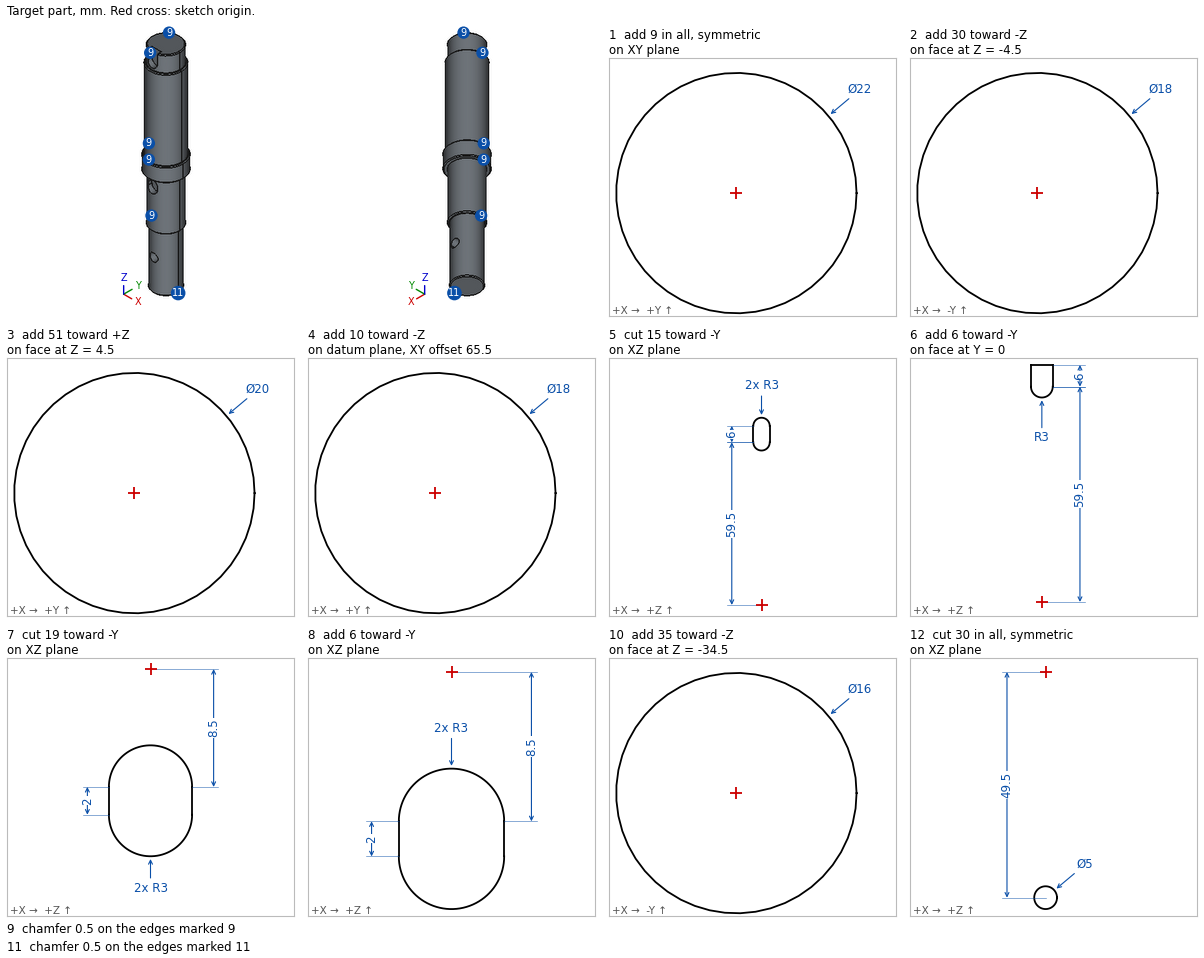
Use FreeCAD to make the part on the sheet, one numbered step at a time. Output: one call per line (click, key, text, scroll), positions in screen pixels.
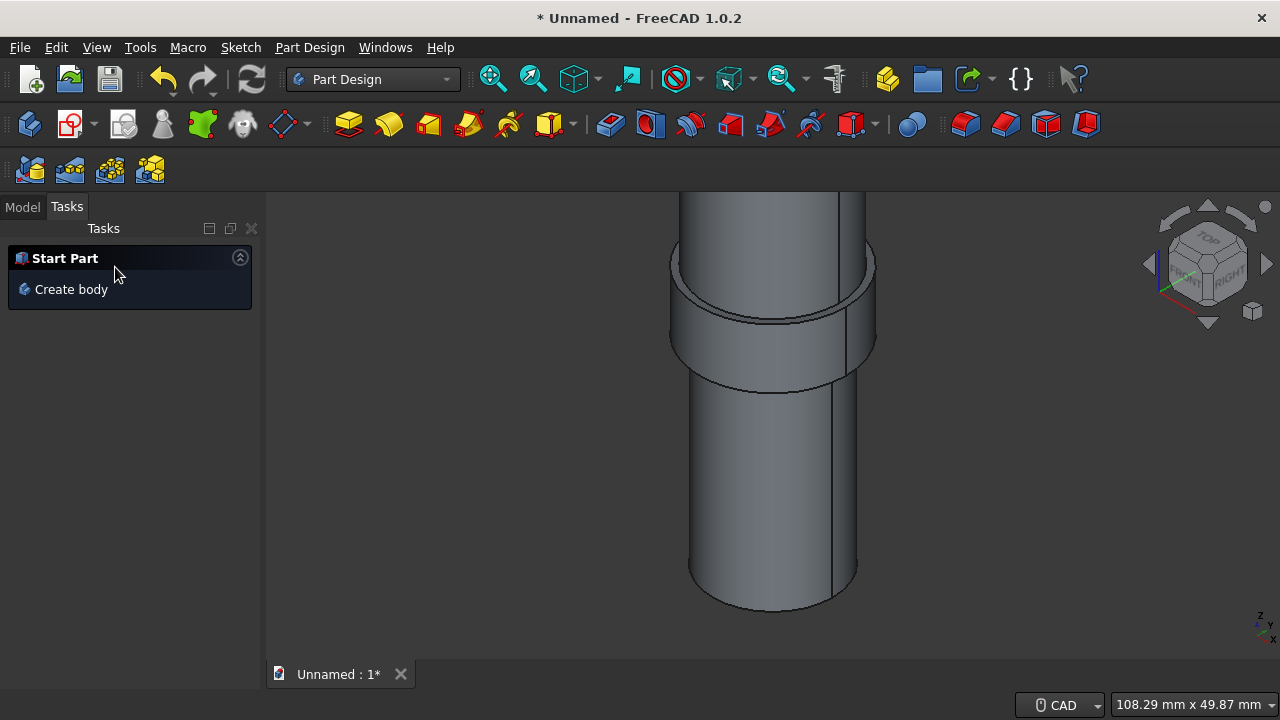
click(494, 80)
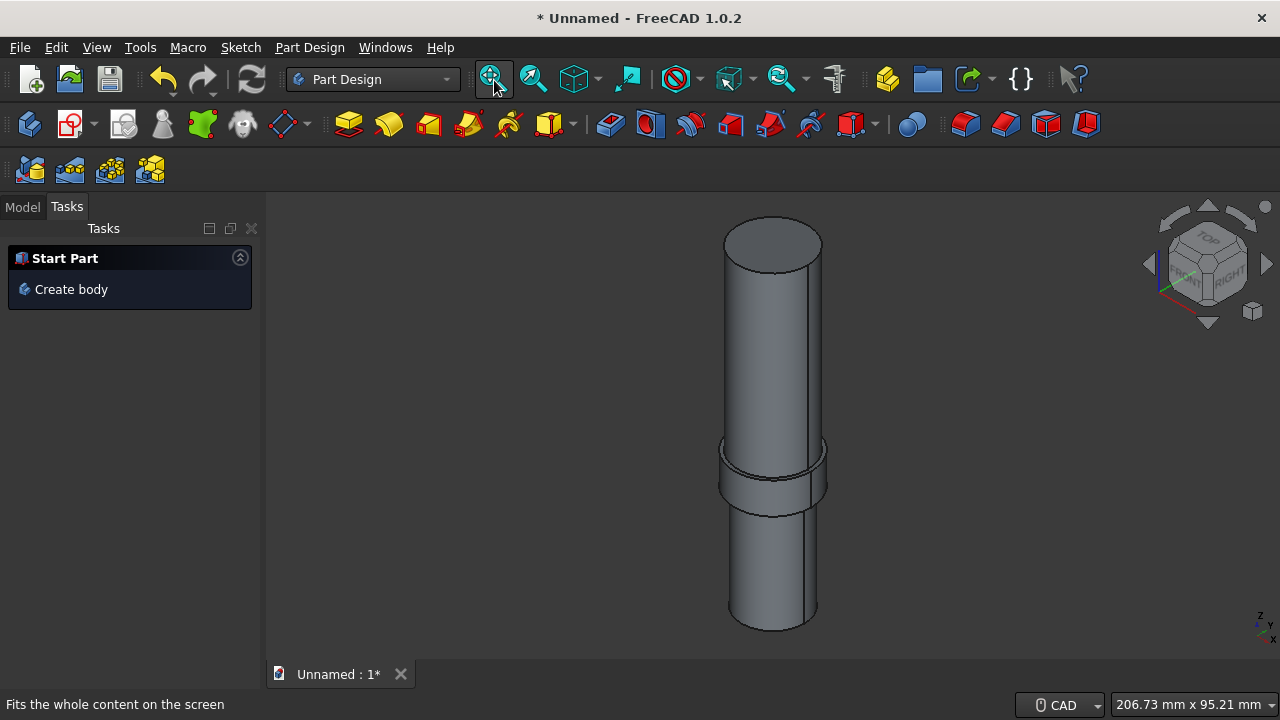
click(23, 206)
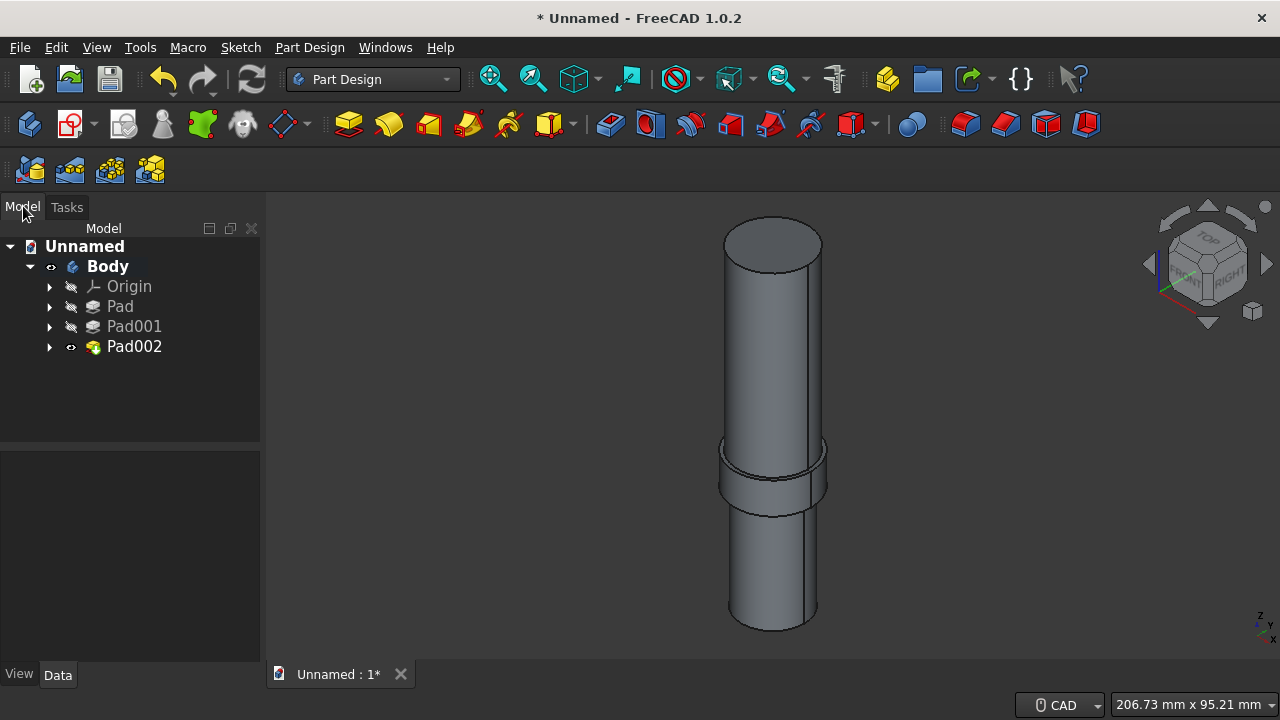
click(50, 287)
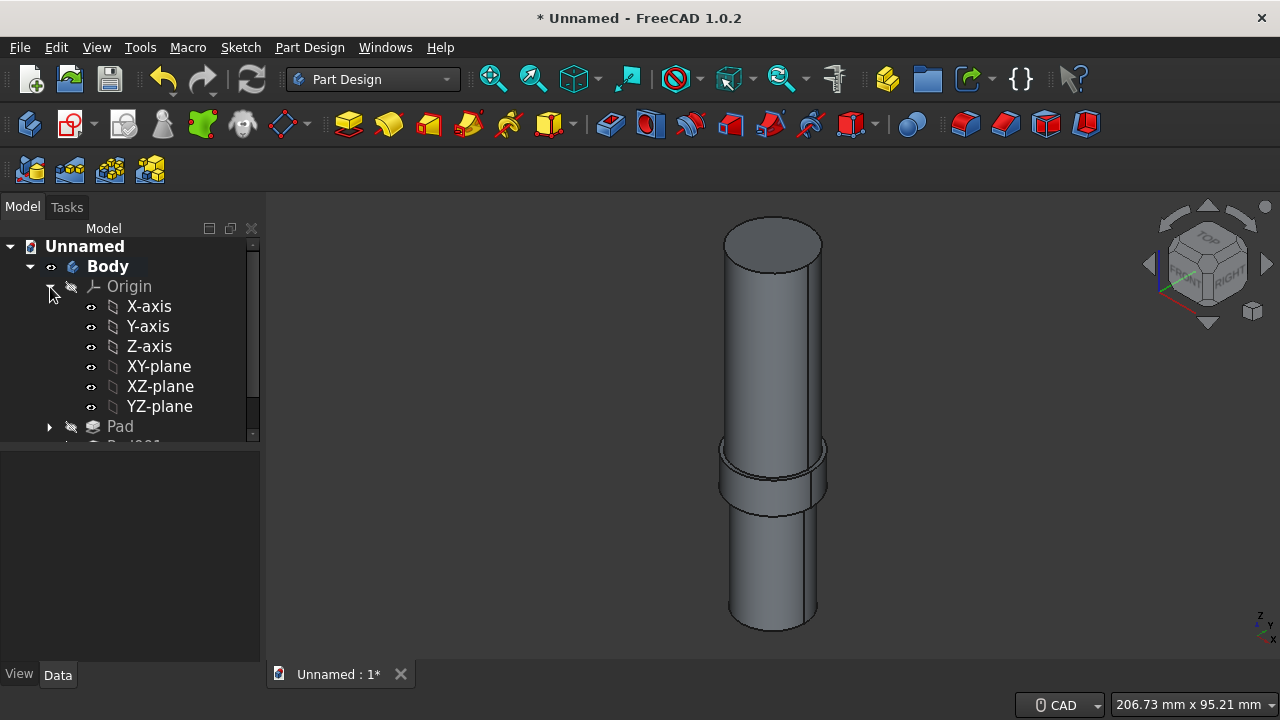
click(136, 367)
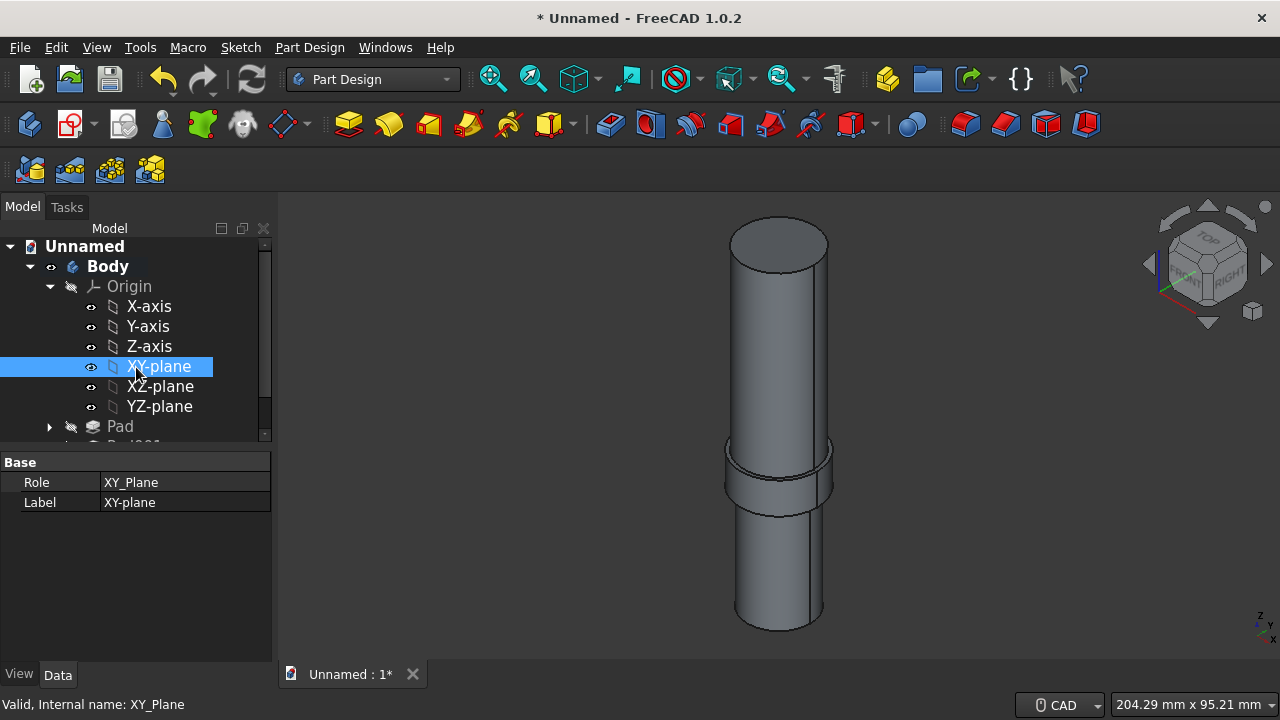
click(284, 124)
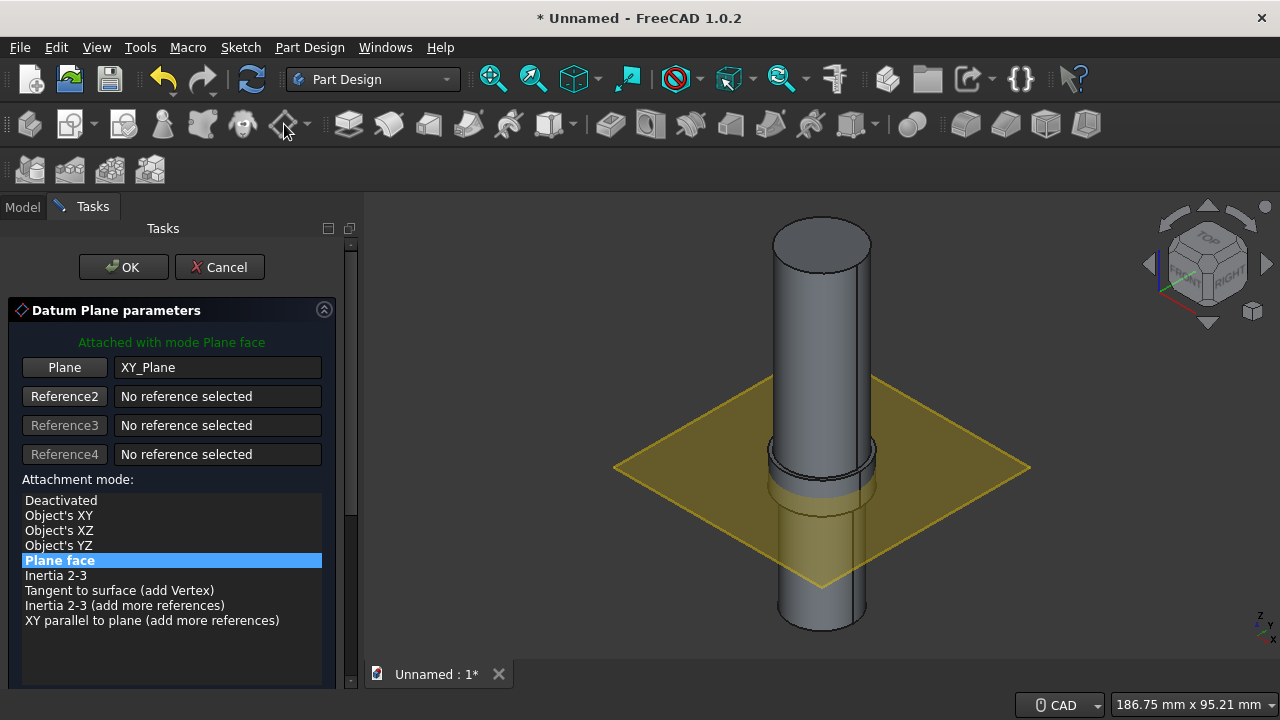
scroll(351, 463, down, 3)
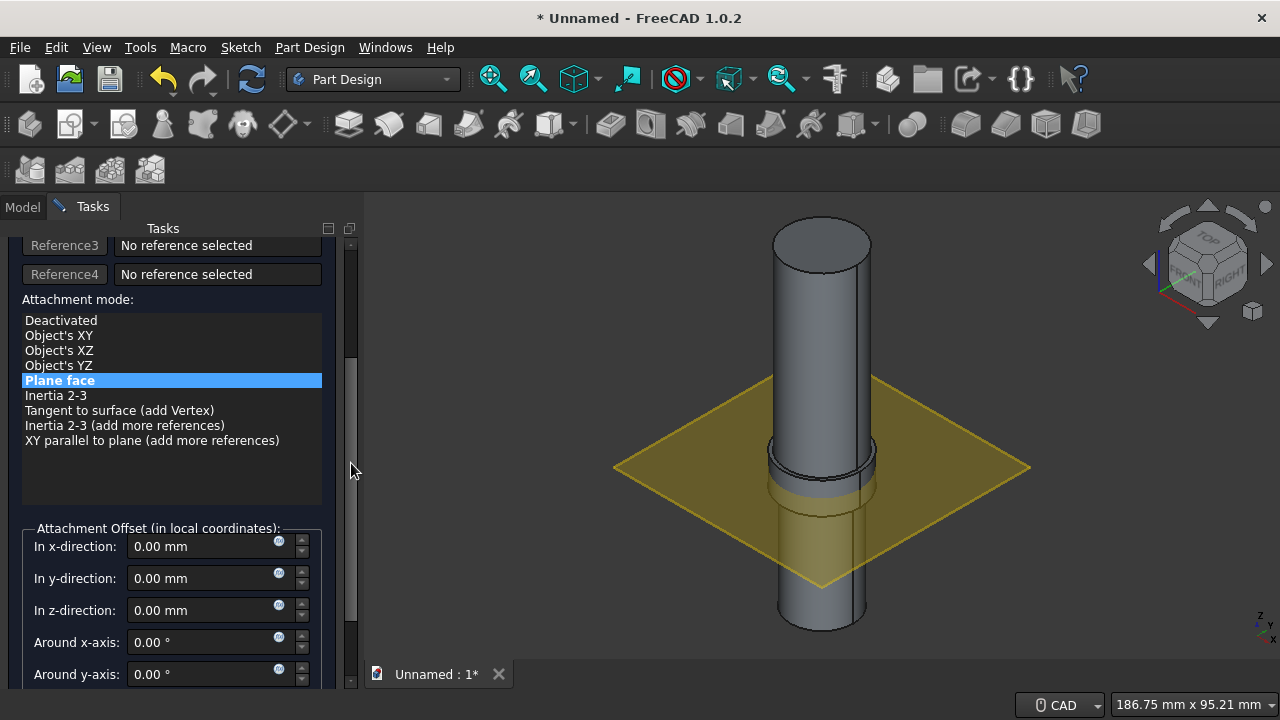
triple_click(210, 610)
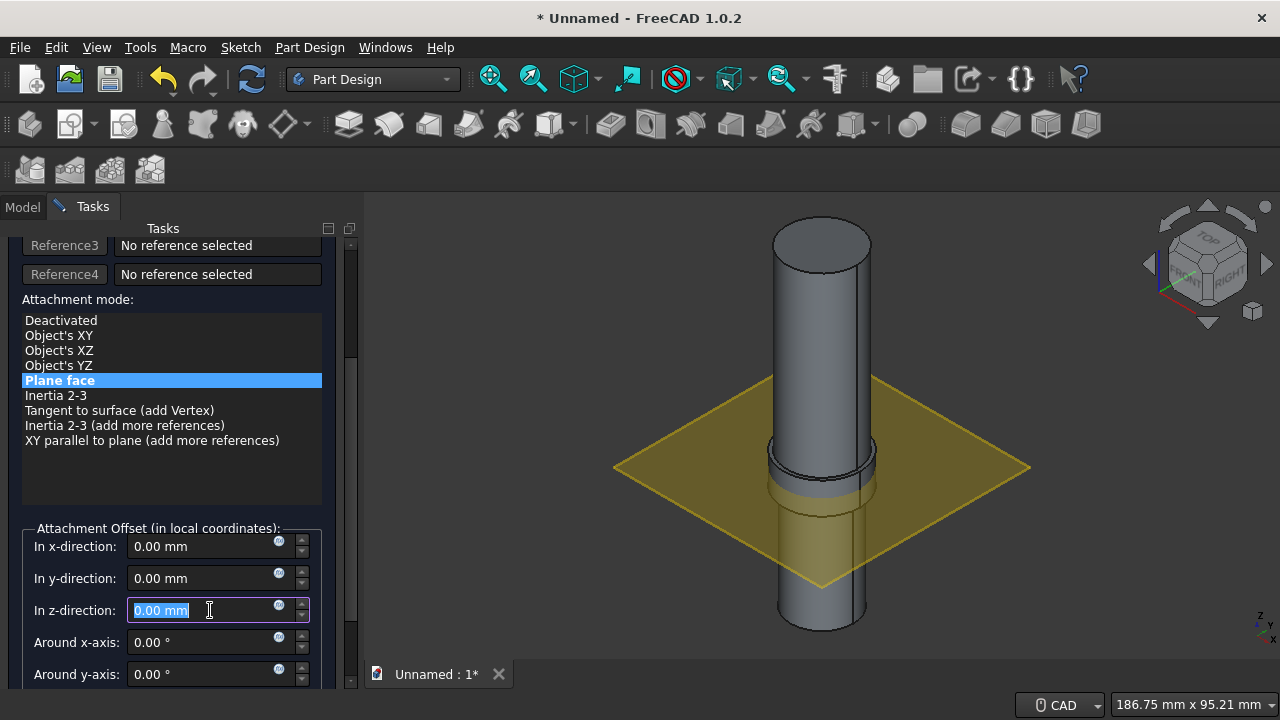
text(65.5)
key(Tab)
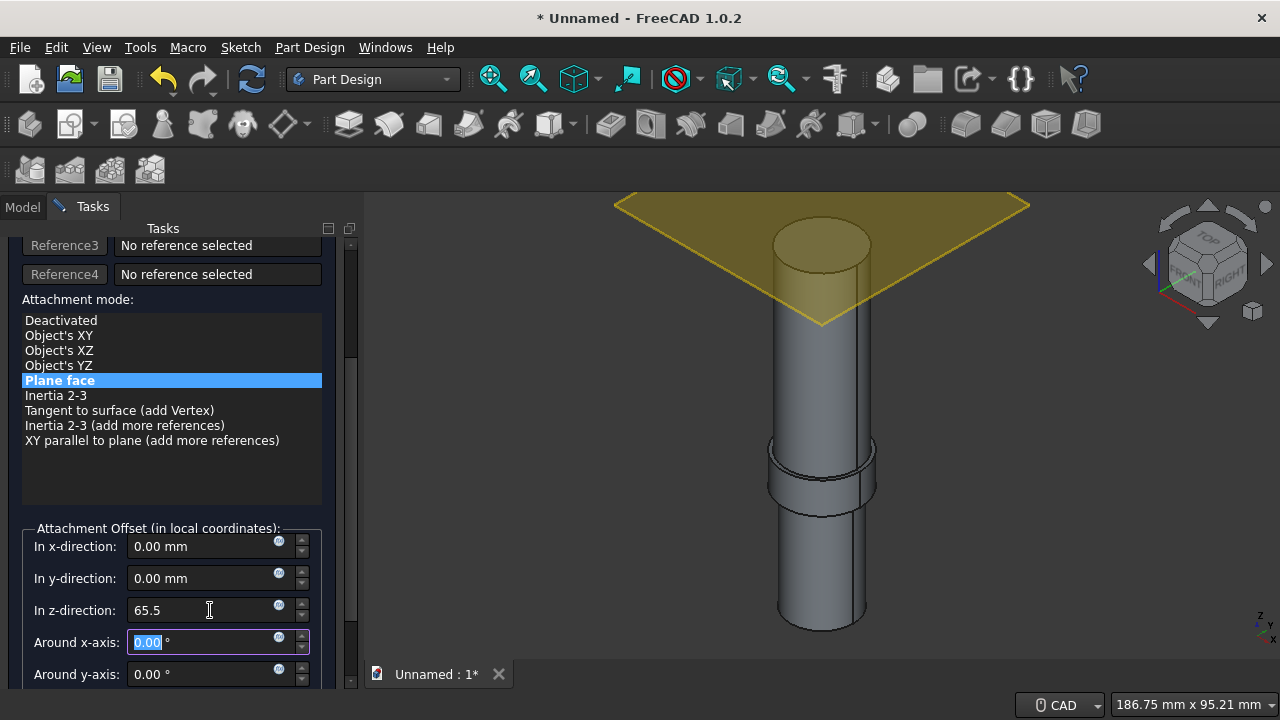
scroll(351, 463, up, 4)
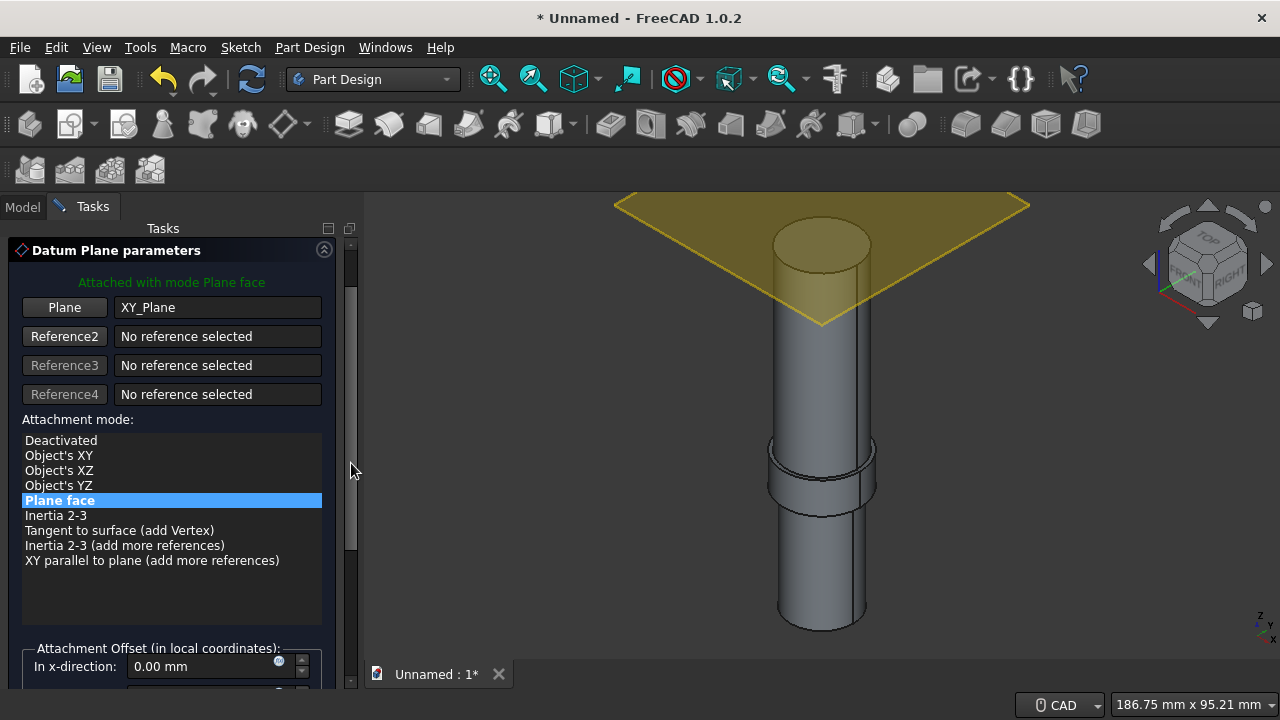
click(124, 267)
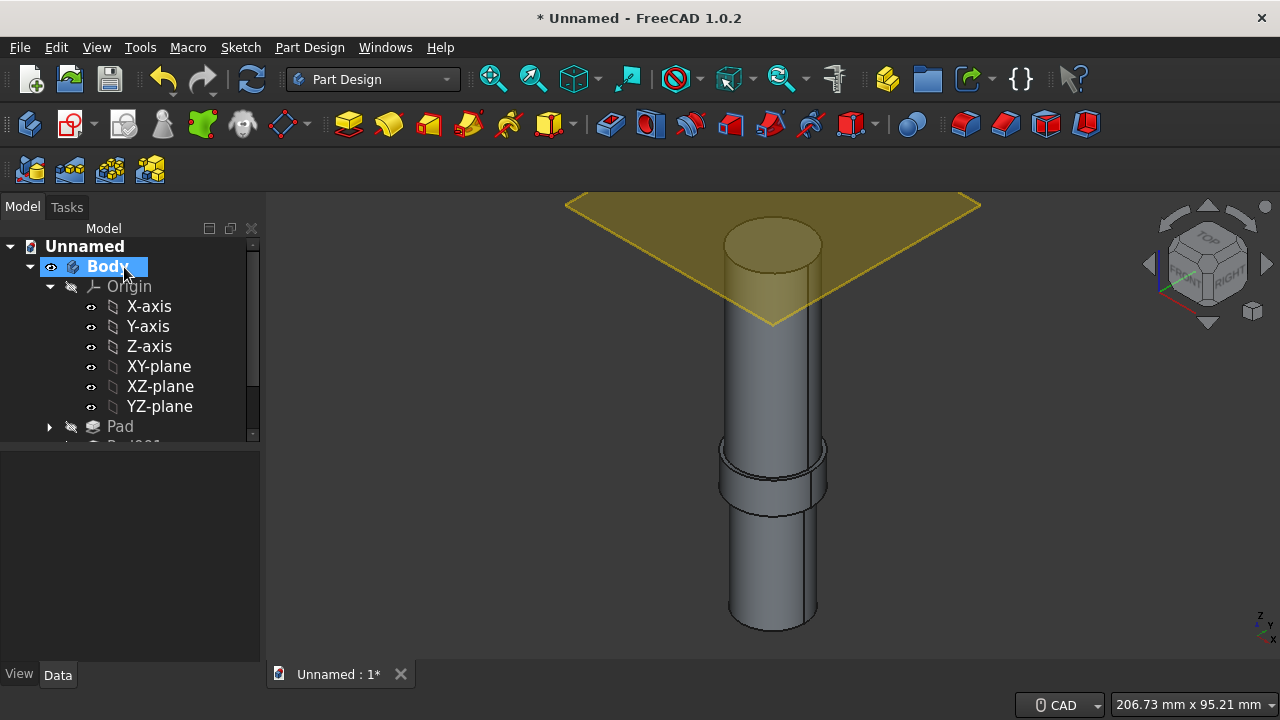
scroll(100, 342, down, 3)